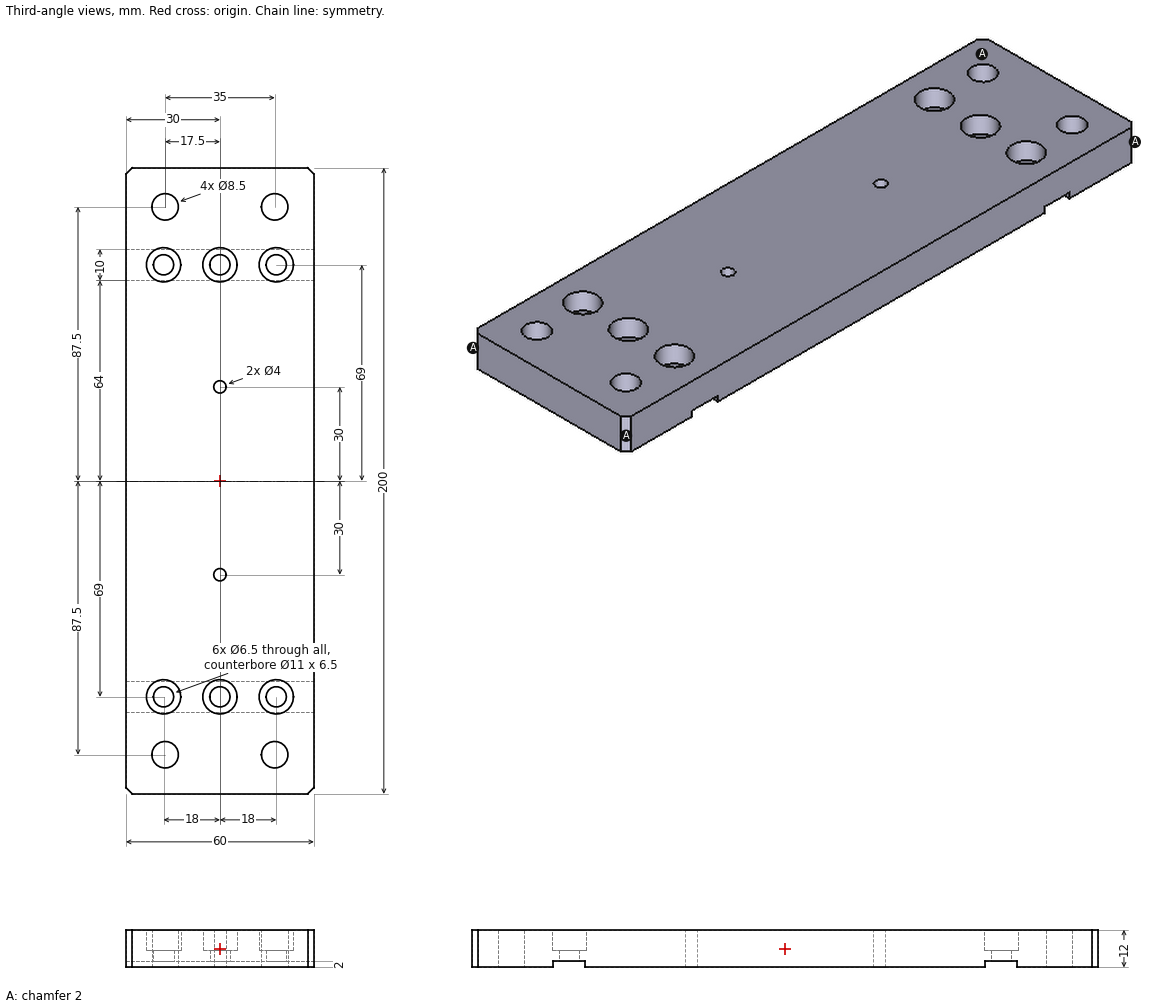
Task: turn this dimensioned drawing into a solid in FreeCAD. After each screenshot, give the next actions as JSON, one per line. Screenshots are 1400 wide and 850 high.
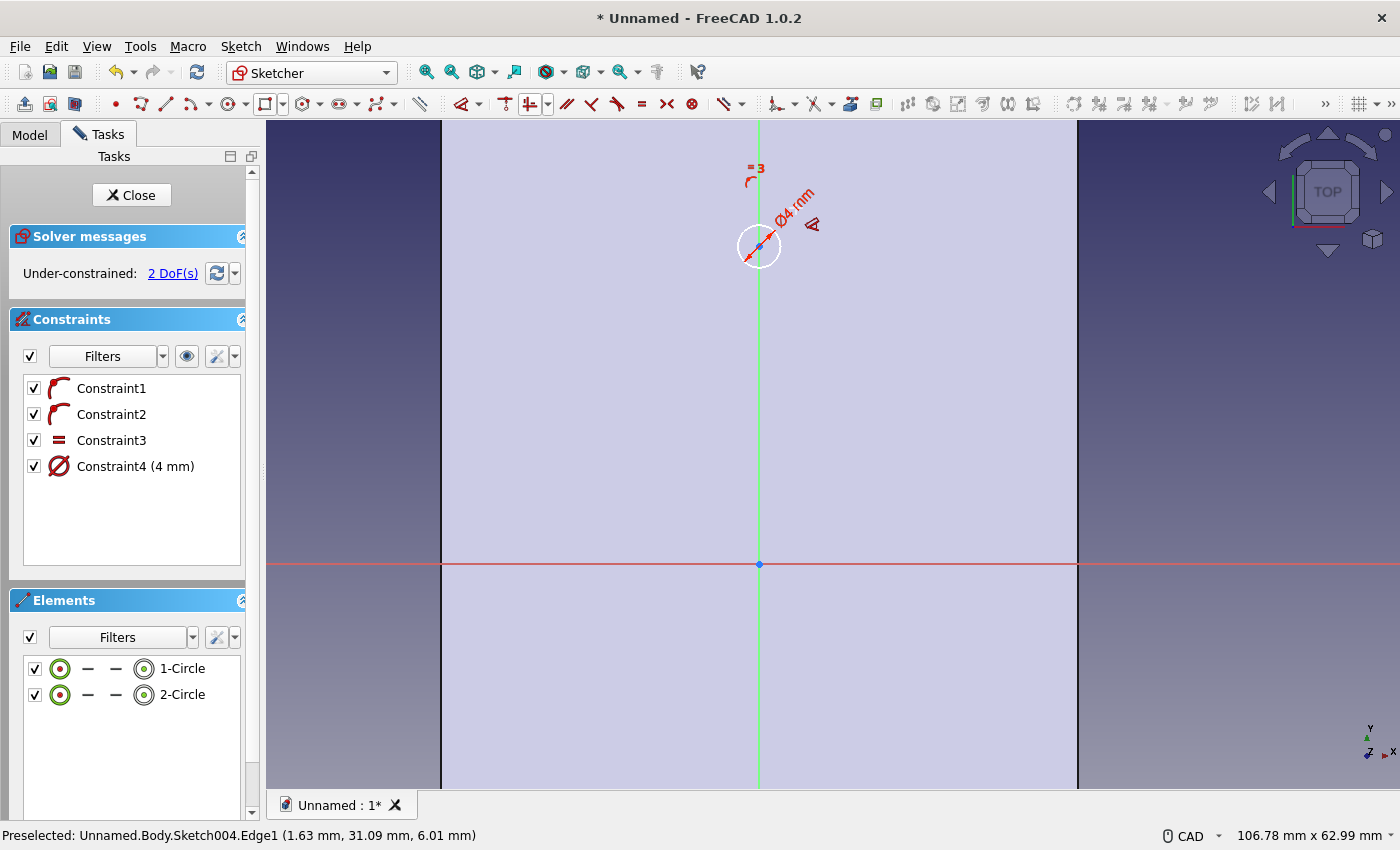
{"action": "left_click", "coordinate": [759, 246]}
{"action": "left_click", "coordinate": [793, 405]}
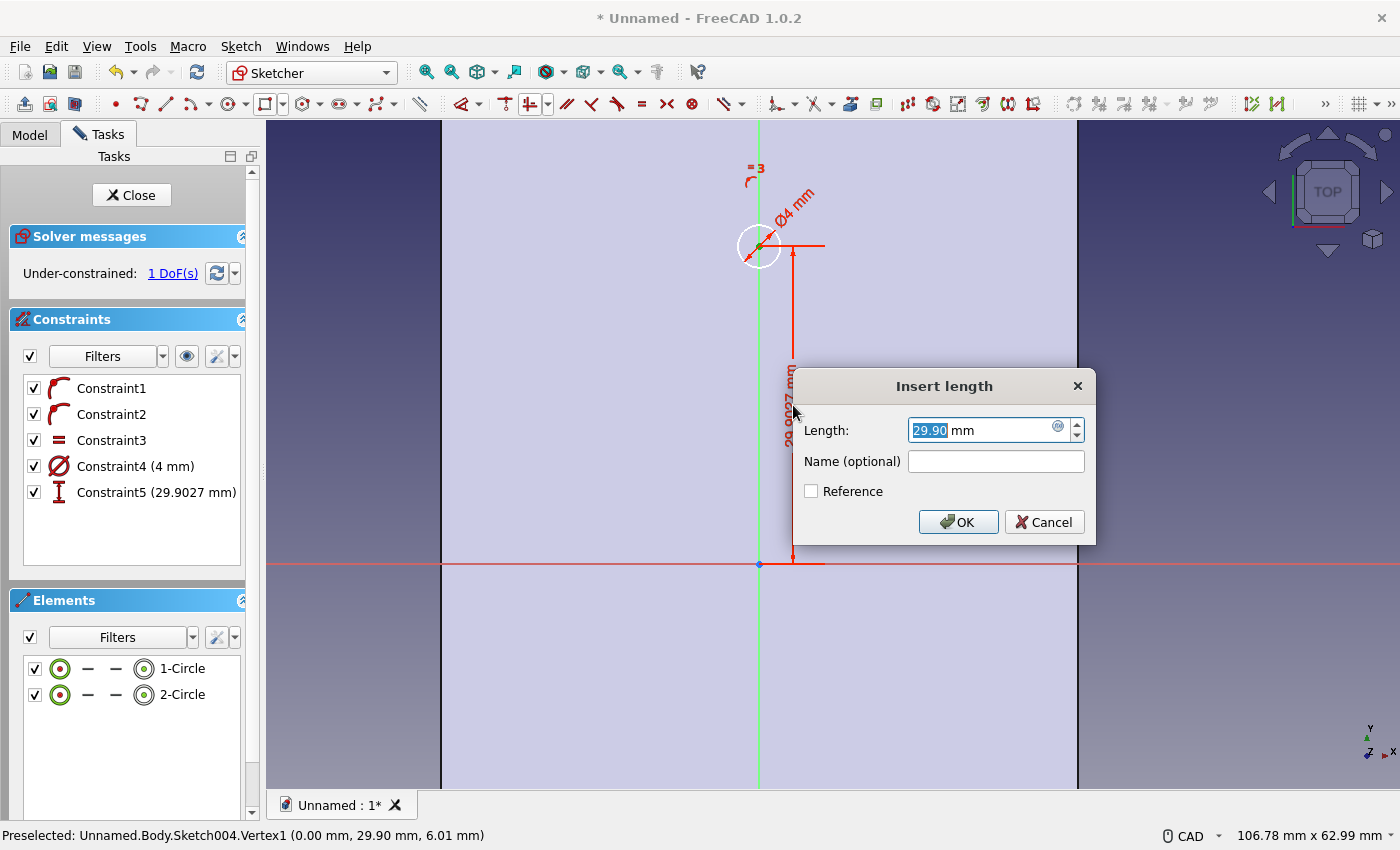
{"action": "type", "text": "30"}
{"action": "key", "text": "Return"}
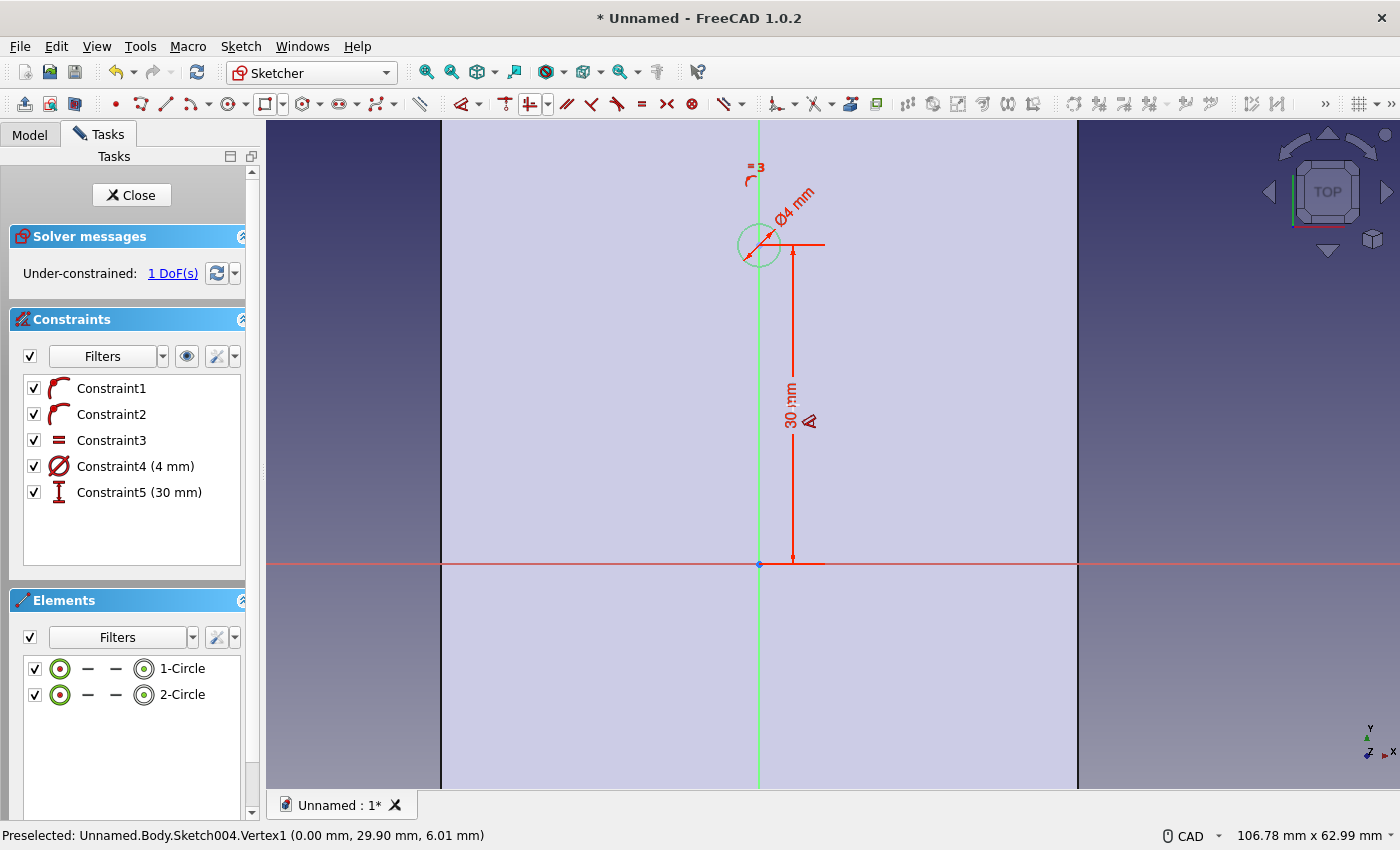
{"action": "scroll", "coordinate": [775, 232], "scroll_direction": "down", "scroll_amount": 2}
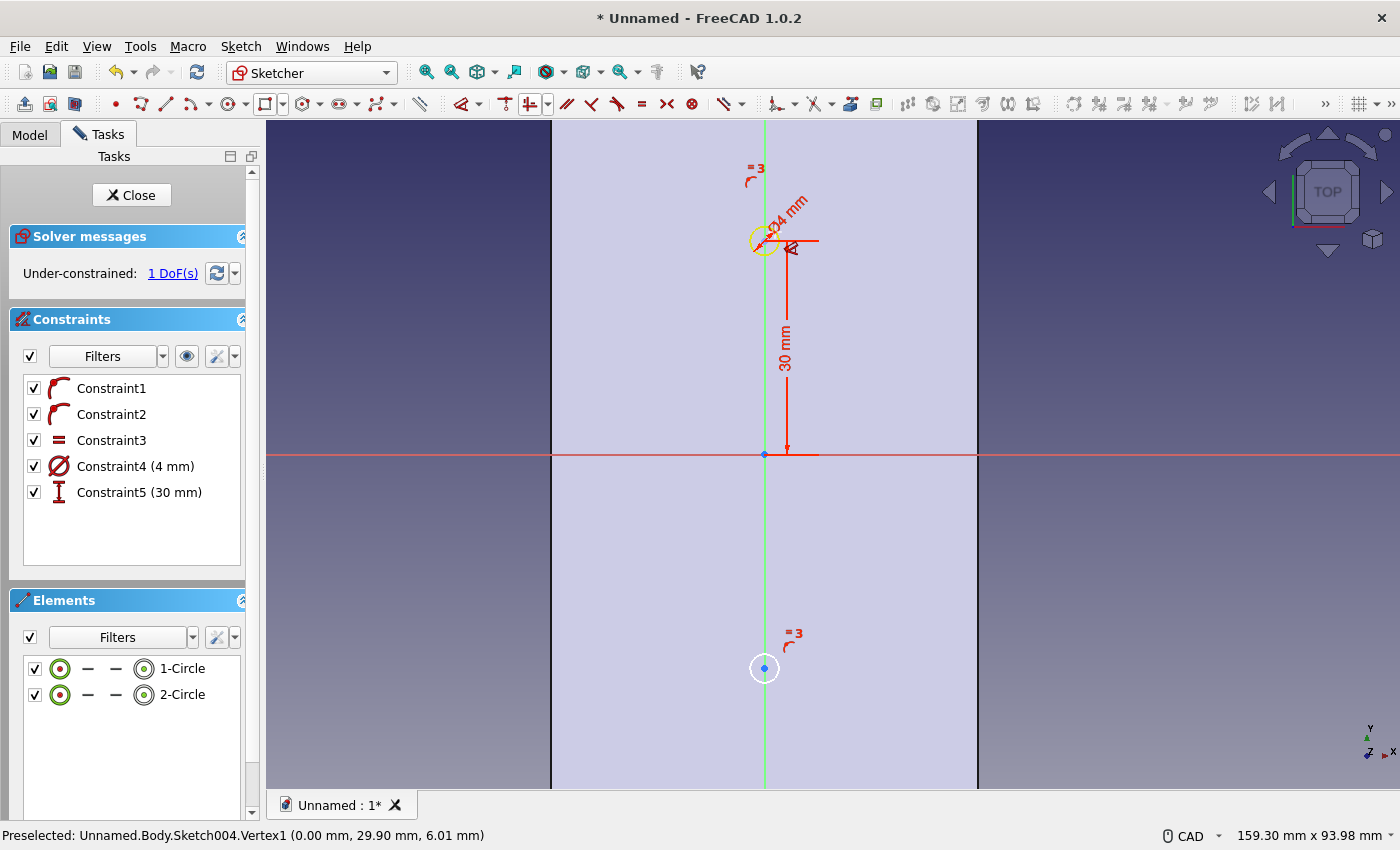
{"action": "left_click", "coordinate": [765, 668]}
{"action": "left_click", "coordinate": [799, 562]}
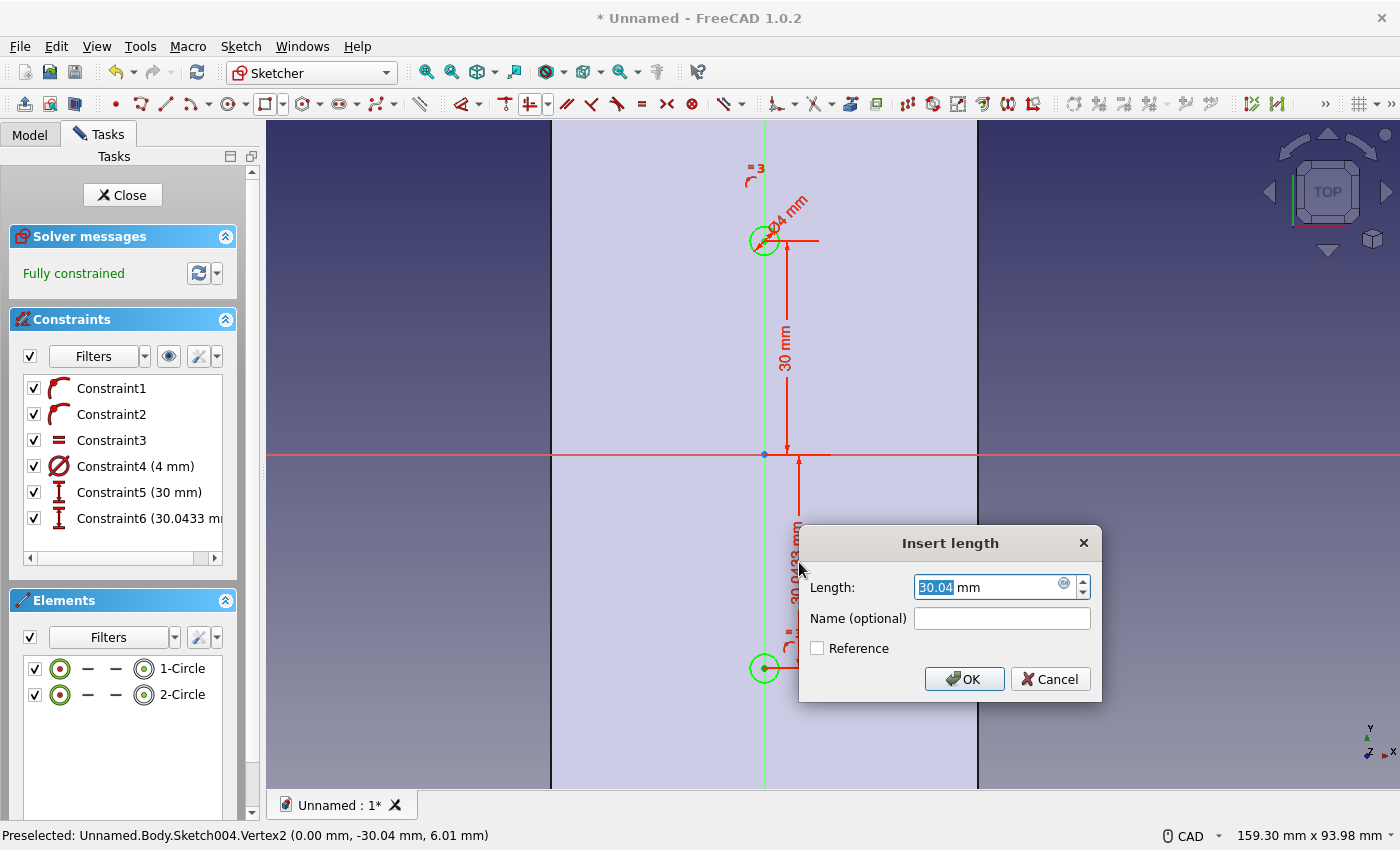
{"action": "type", "text": "30"}
{"action": "key", "text": "Return"}
{"action": "key", "text": "Escape"}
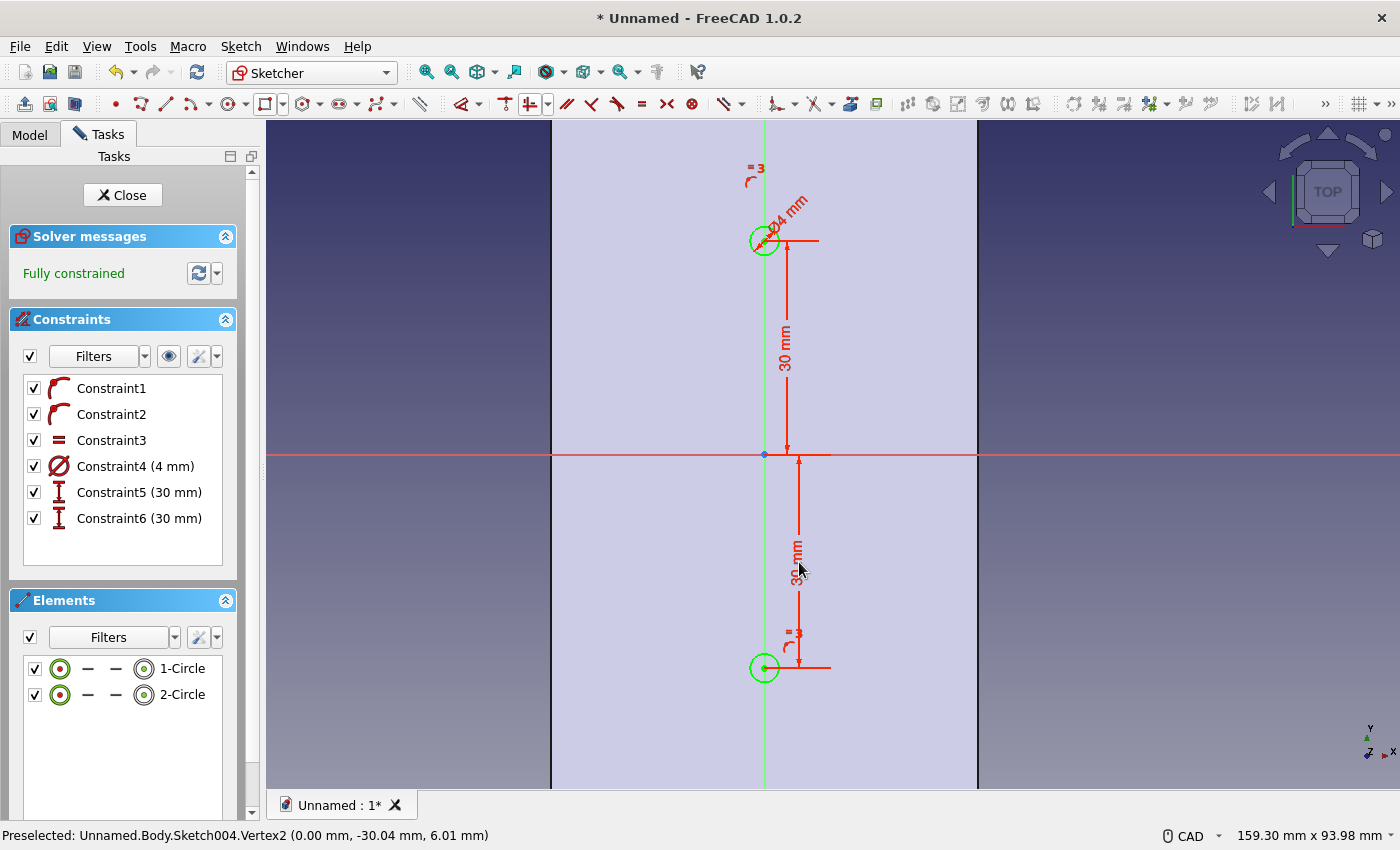
{"action": "left_click", "coordinate": [123, 195]}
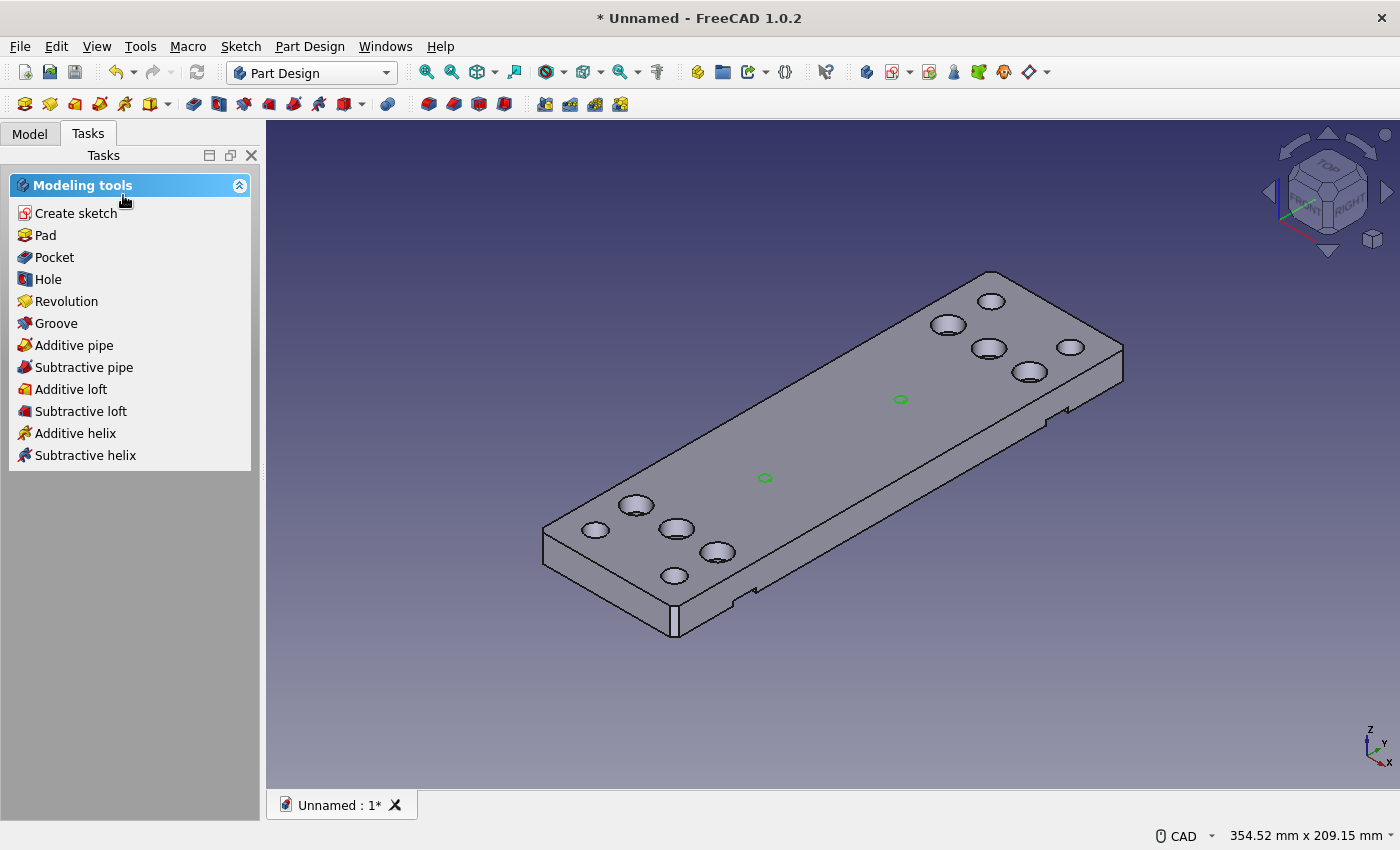
{"action": "left_click", "coordinate": [194, 104]}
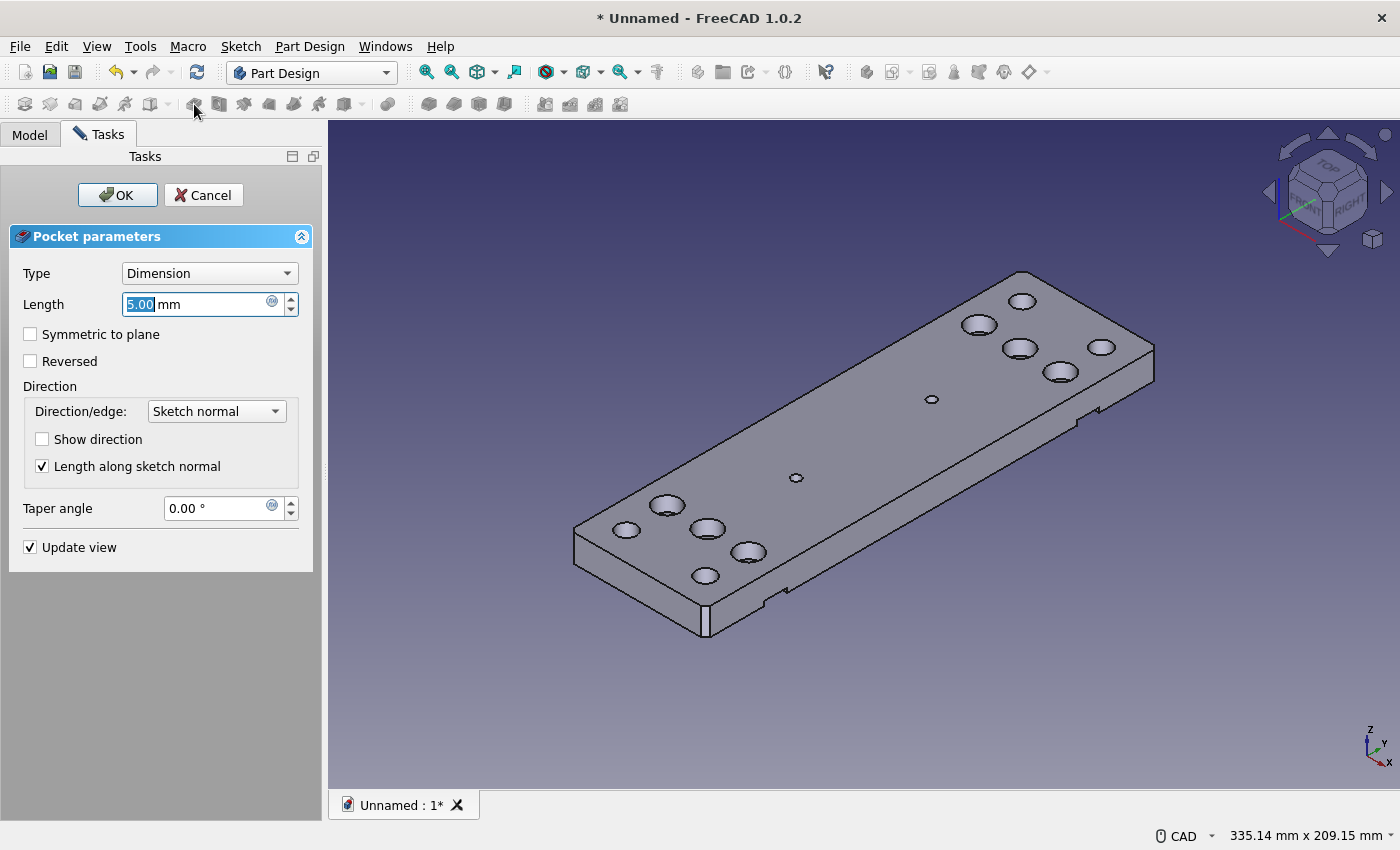
{"action": "left_click", "coordinate": [210, 274]}